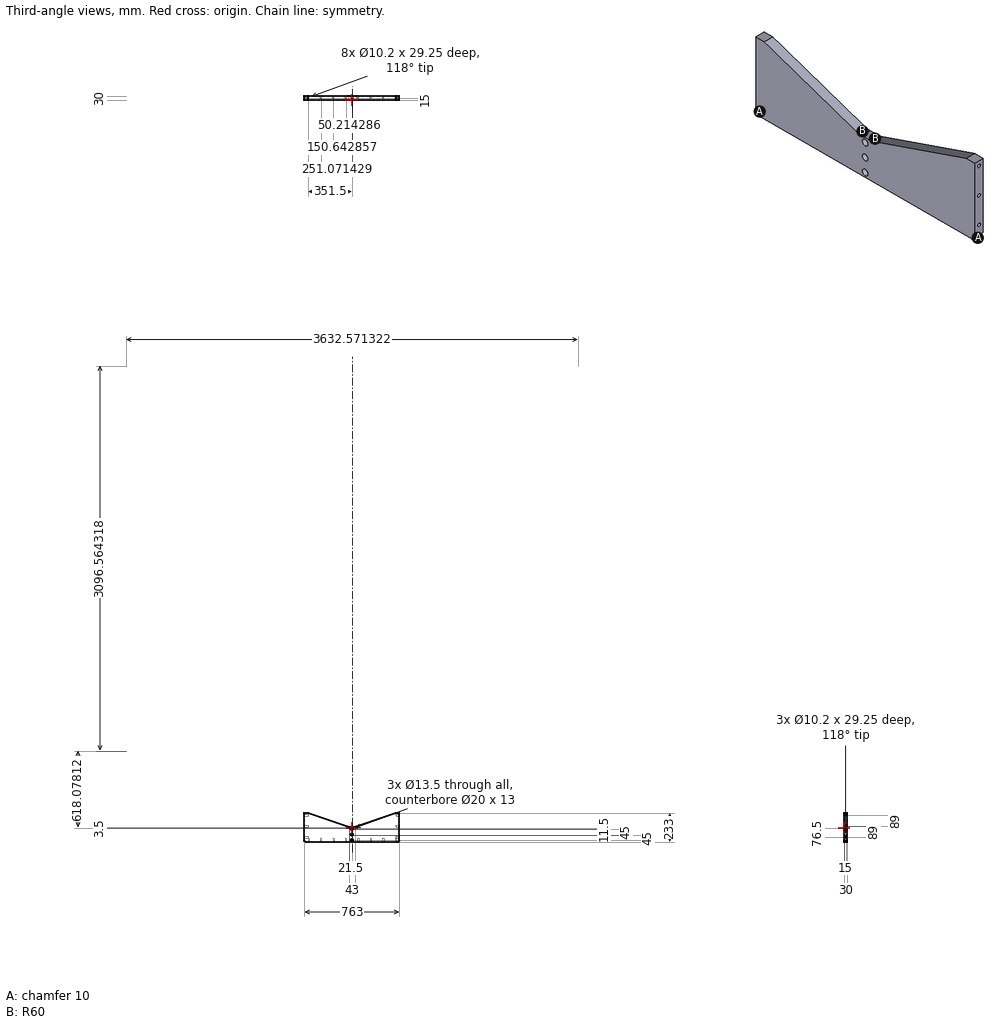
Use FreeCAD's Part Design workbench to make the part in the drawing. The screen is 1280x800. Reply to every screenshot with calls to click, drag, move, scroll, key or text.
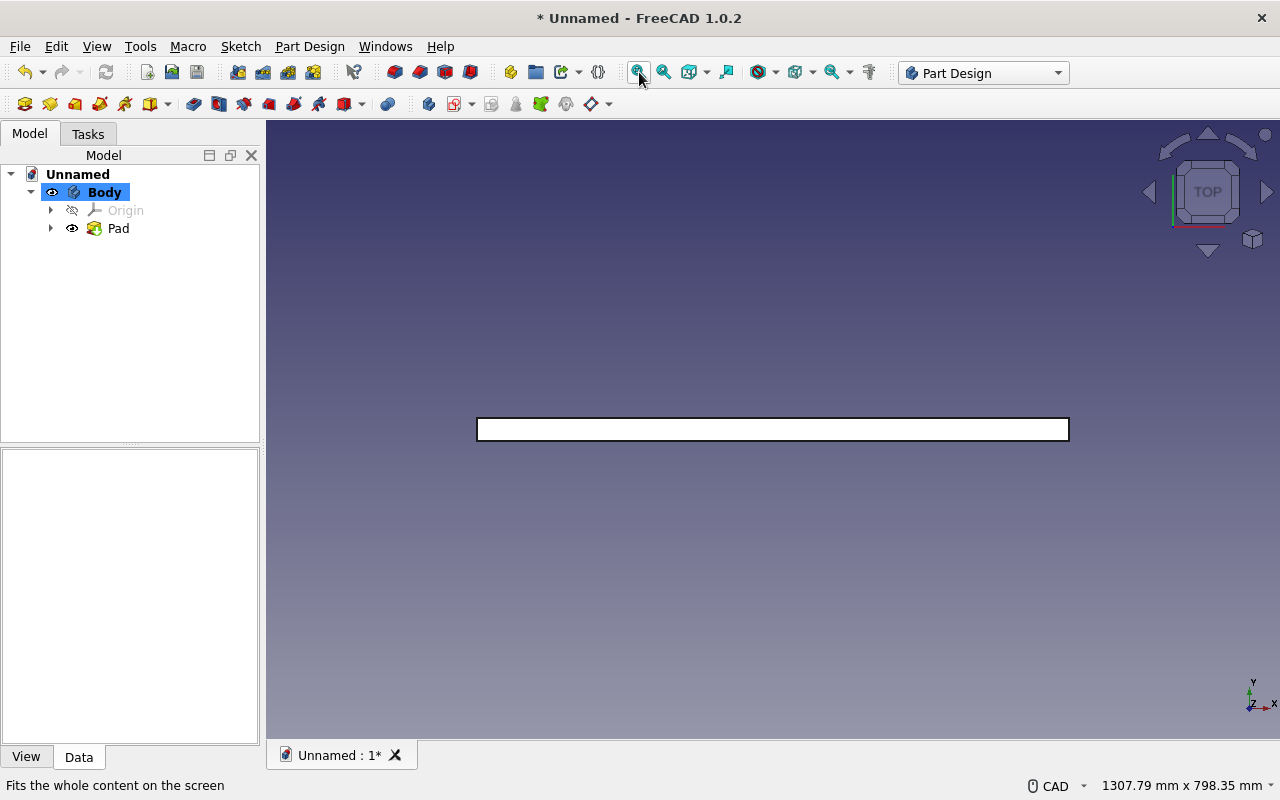
key(1)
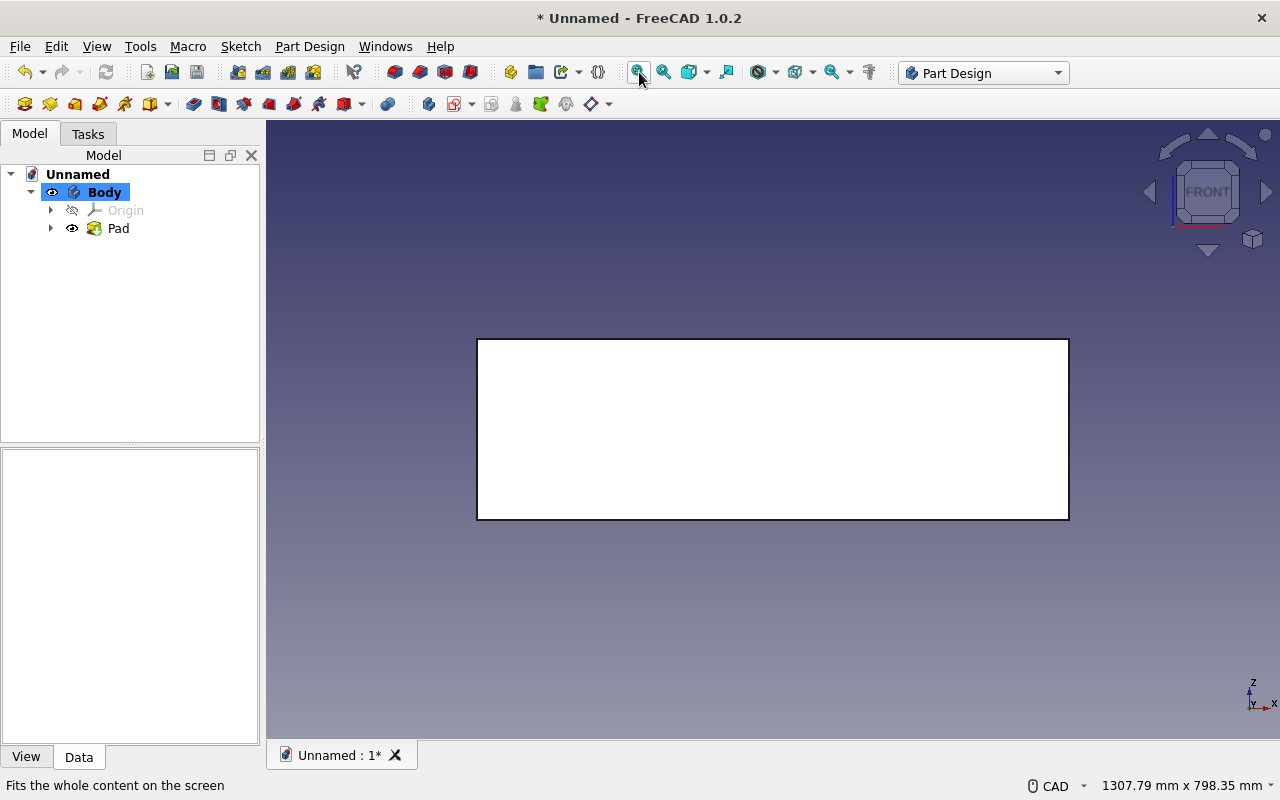
key(3)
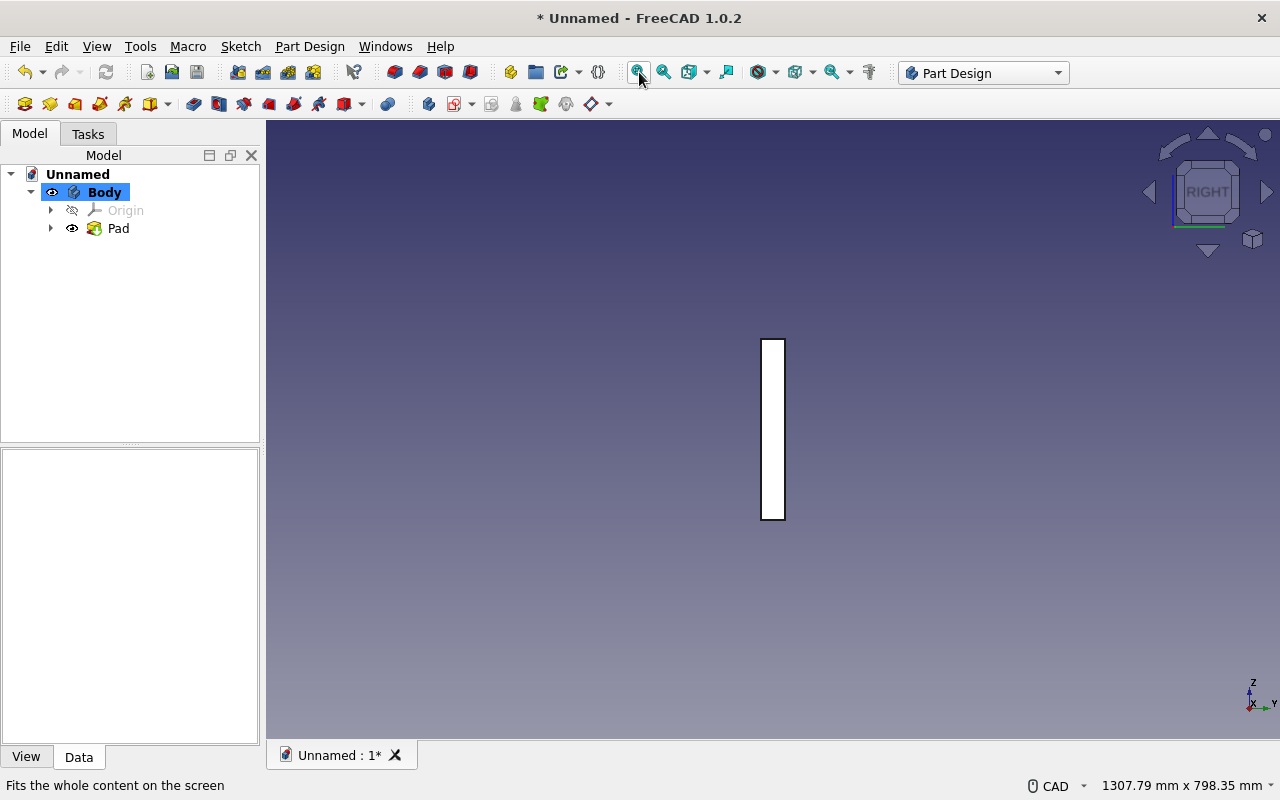
click(639, 72)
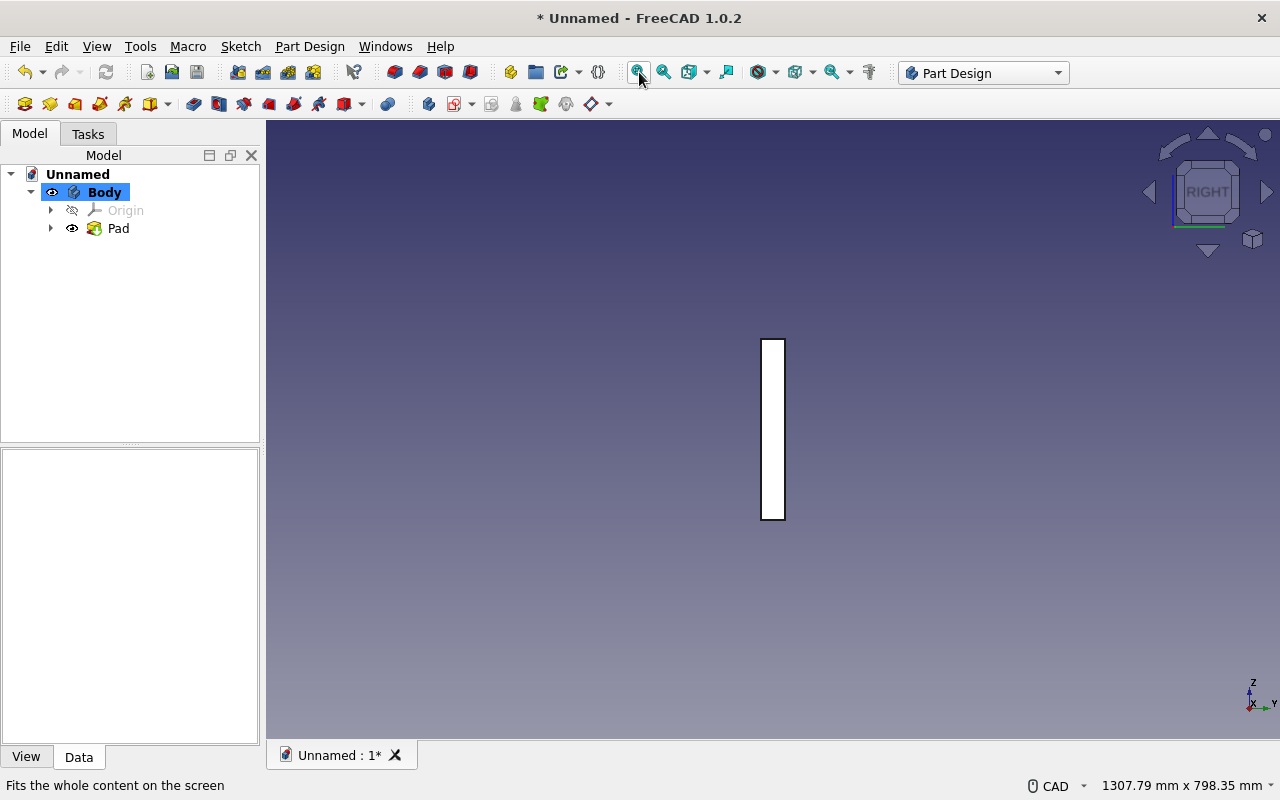
click(773, 519)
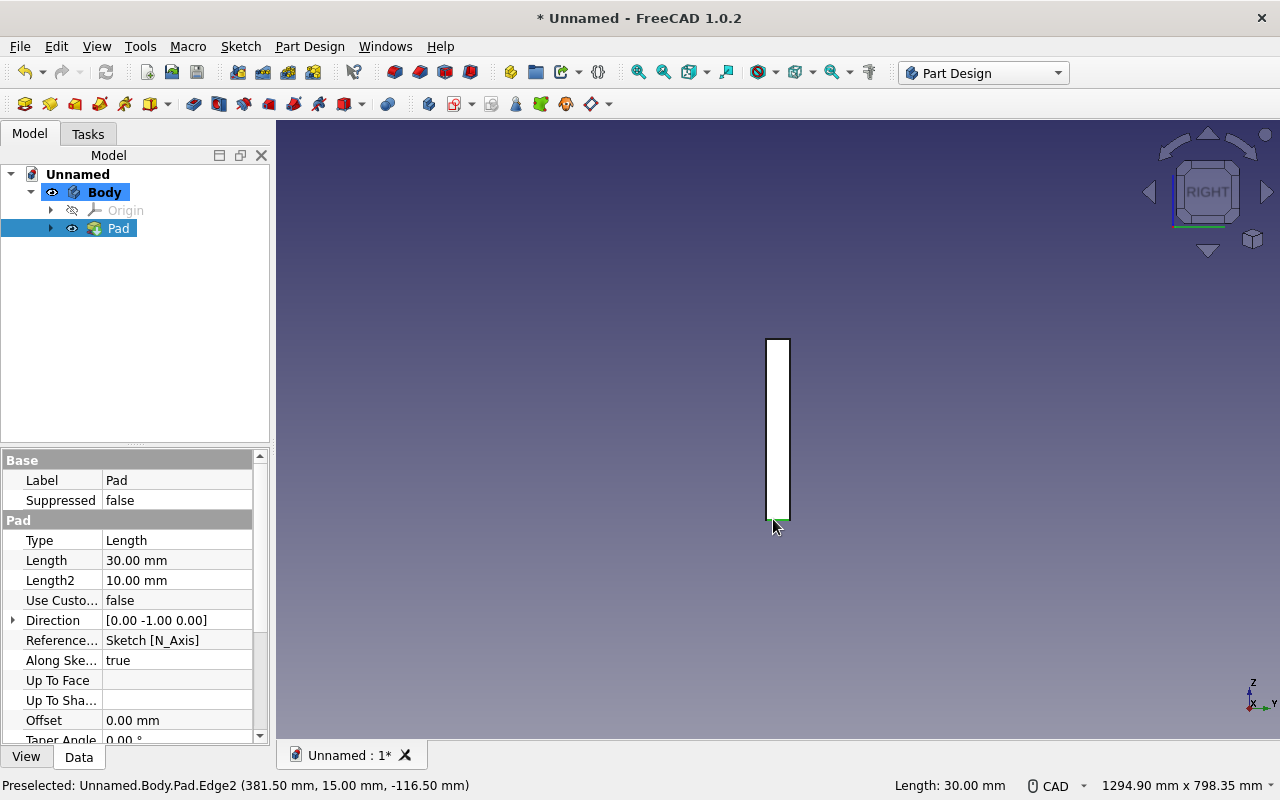
key(5)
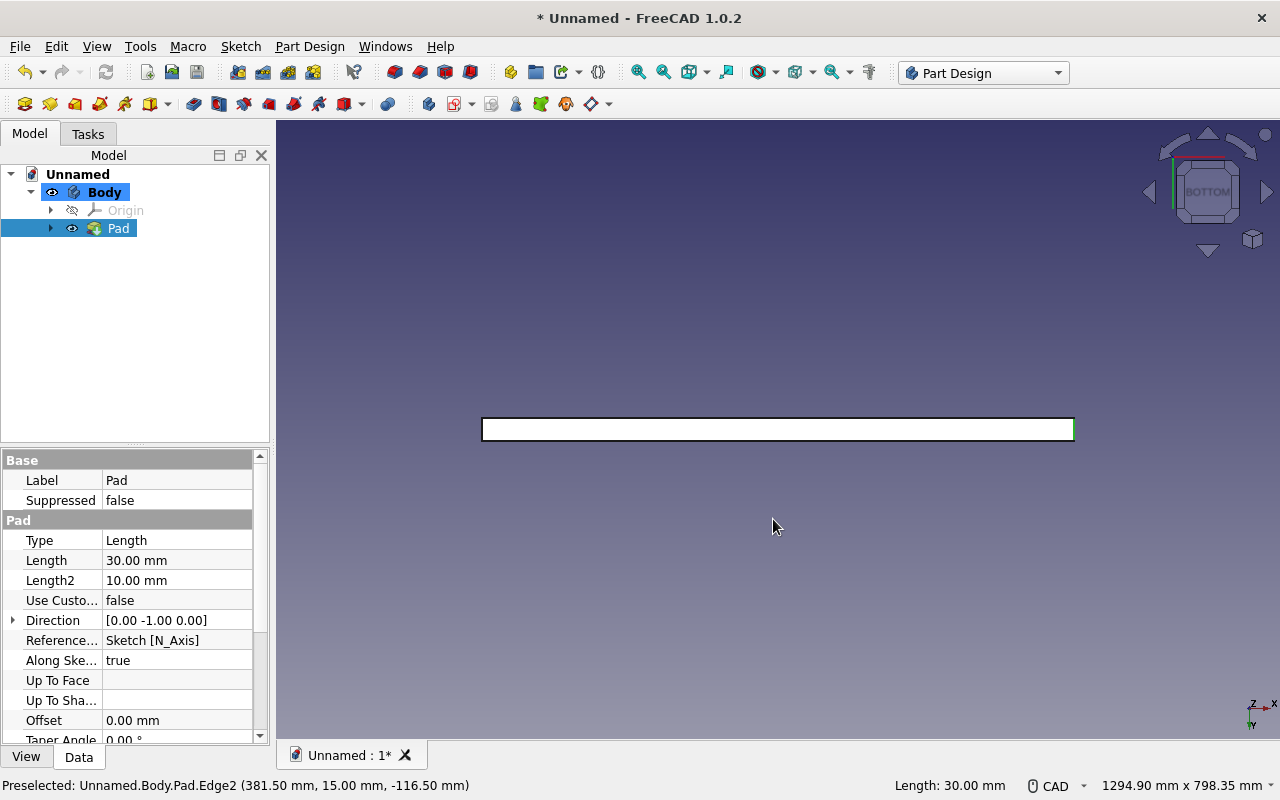
click(482, 428, ctrl)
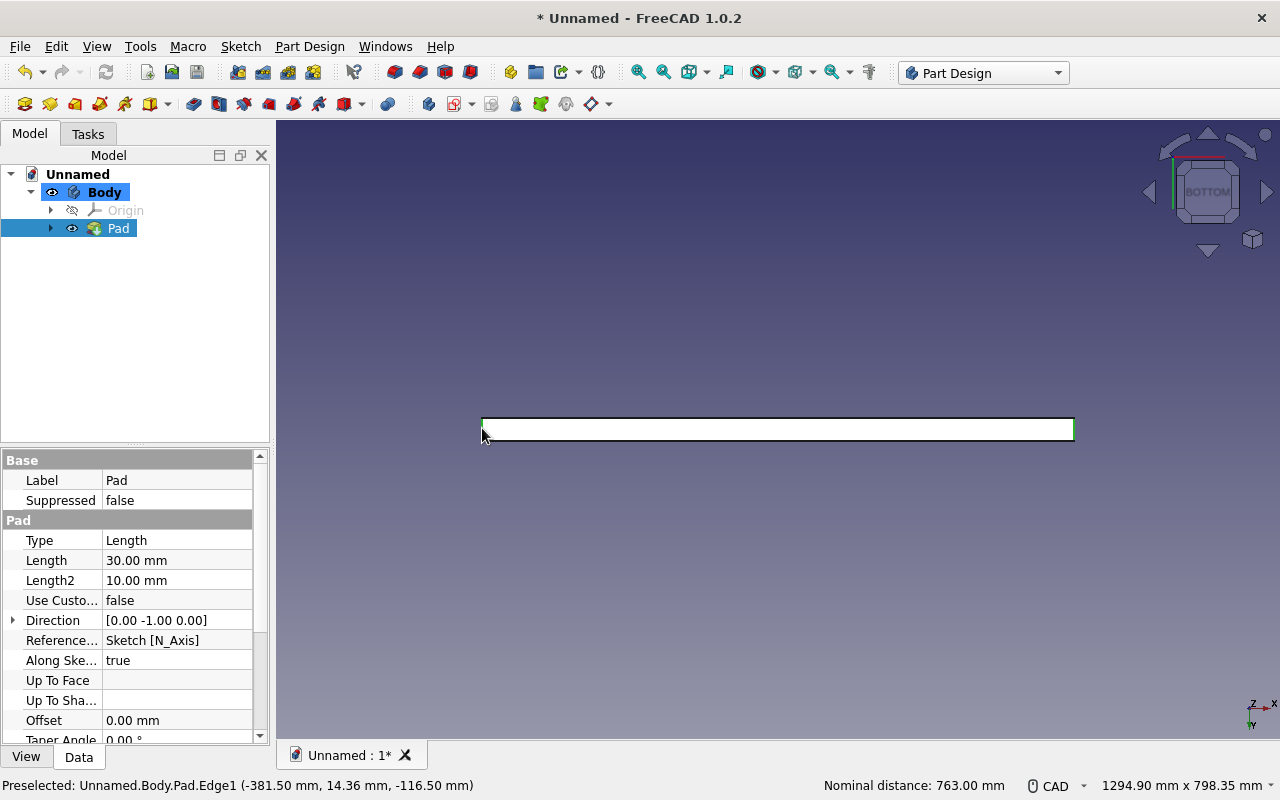
click(420, 72)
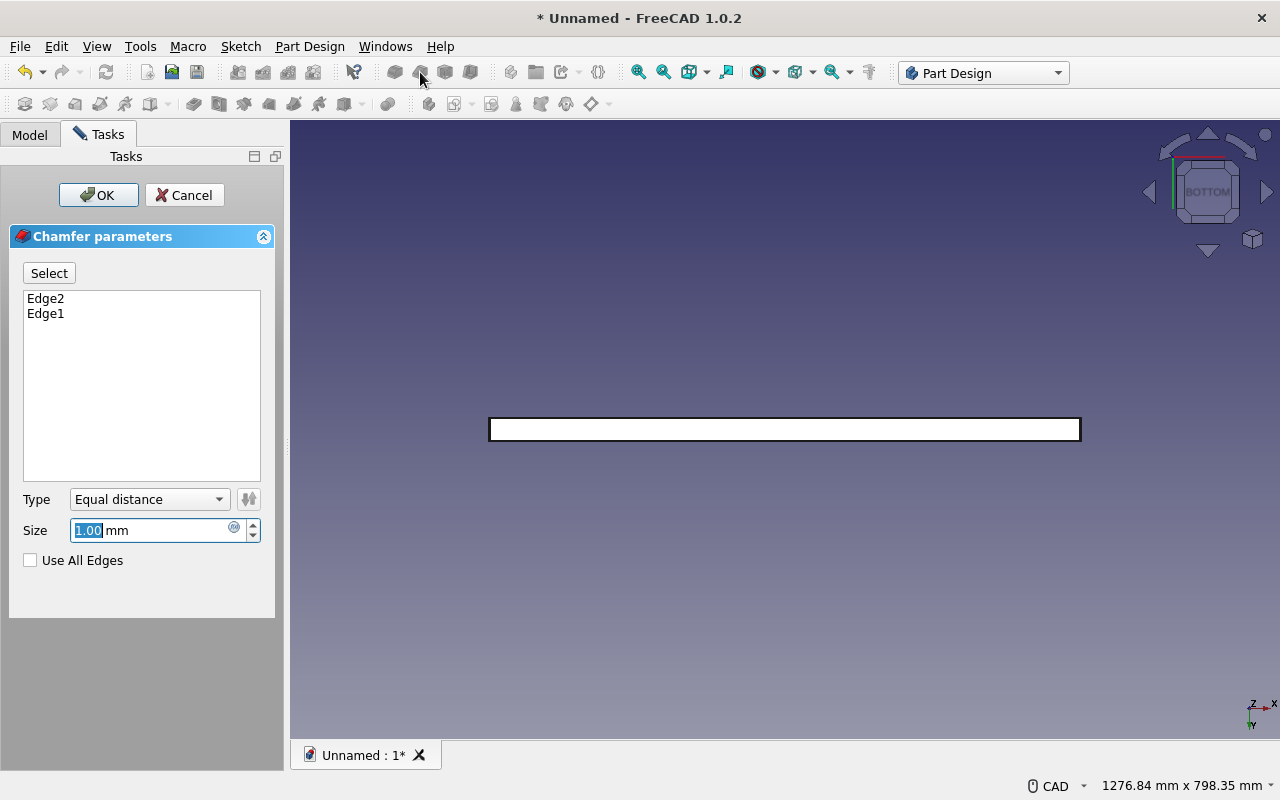
text(10)
key(Tab)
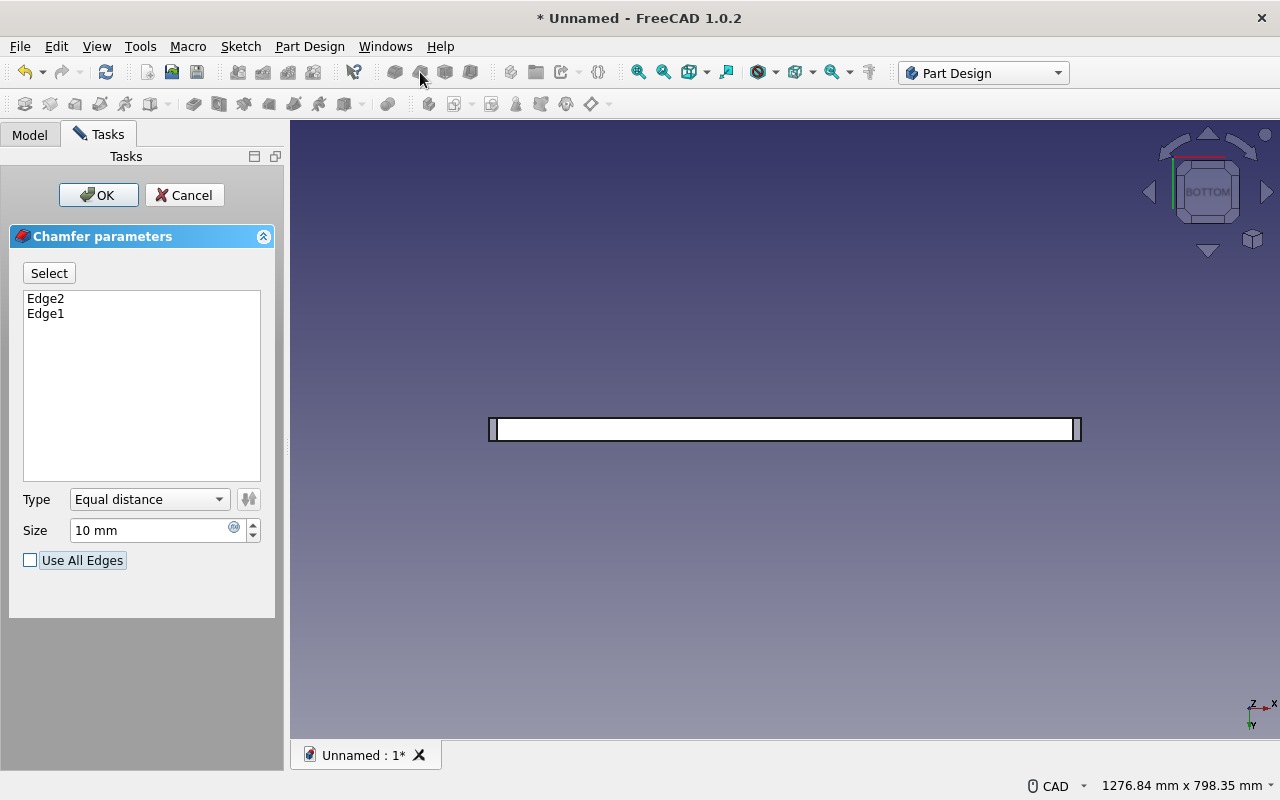
click(99, 195)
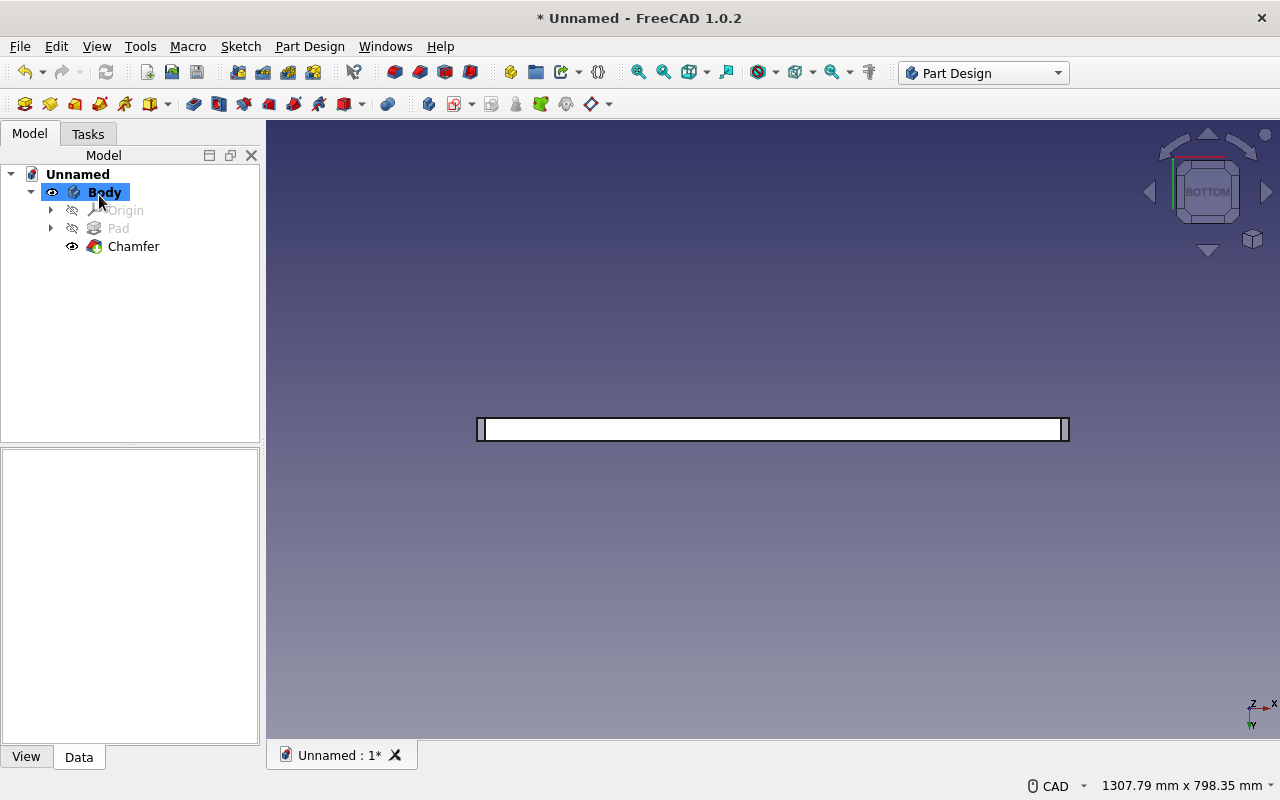
key(4)